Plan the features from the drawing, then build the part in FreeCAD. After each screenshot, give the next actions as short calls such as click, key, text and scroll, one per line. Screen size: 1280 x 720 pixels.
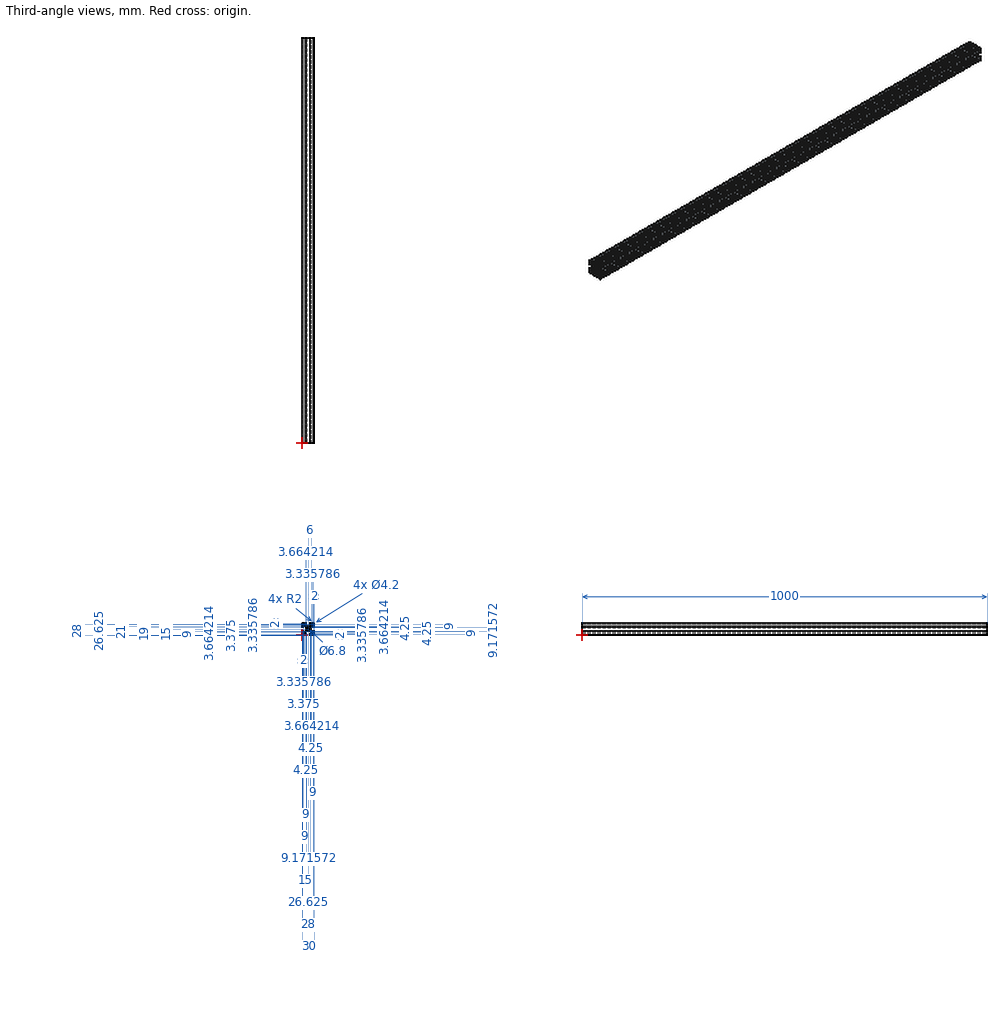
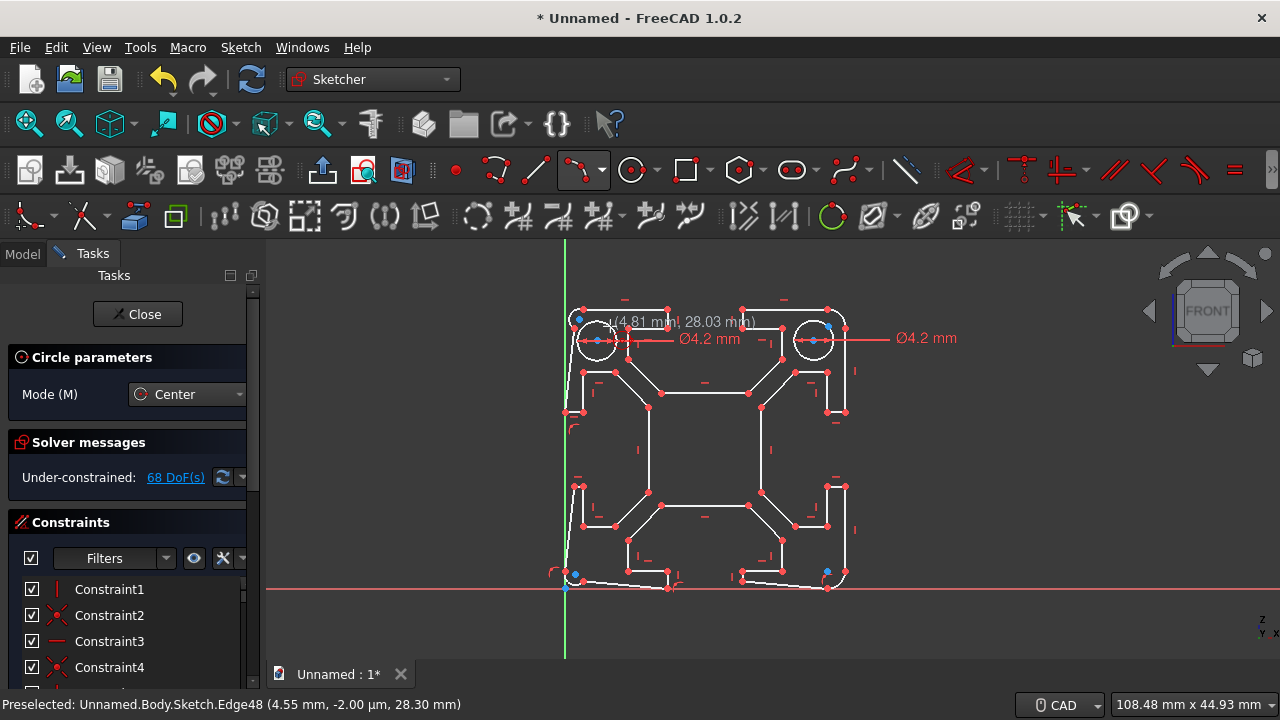
click(814, 557)
move(828, 544)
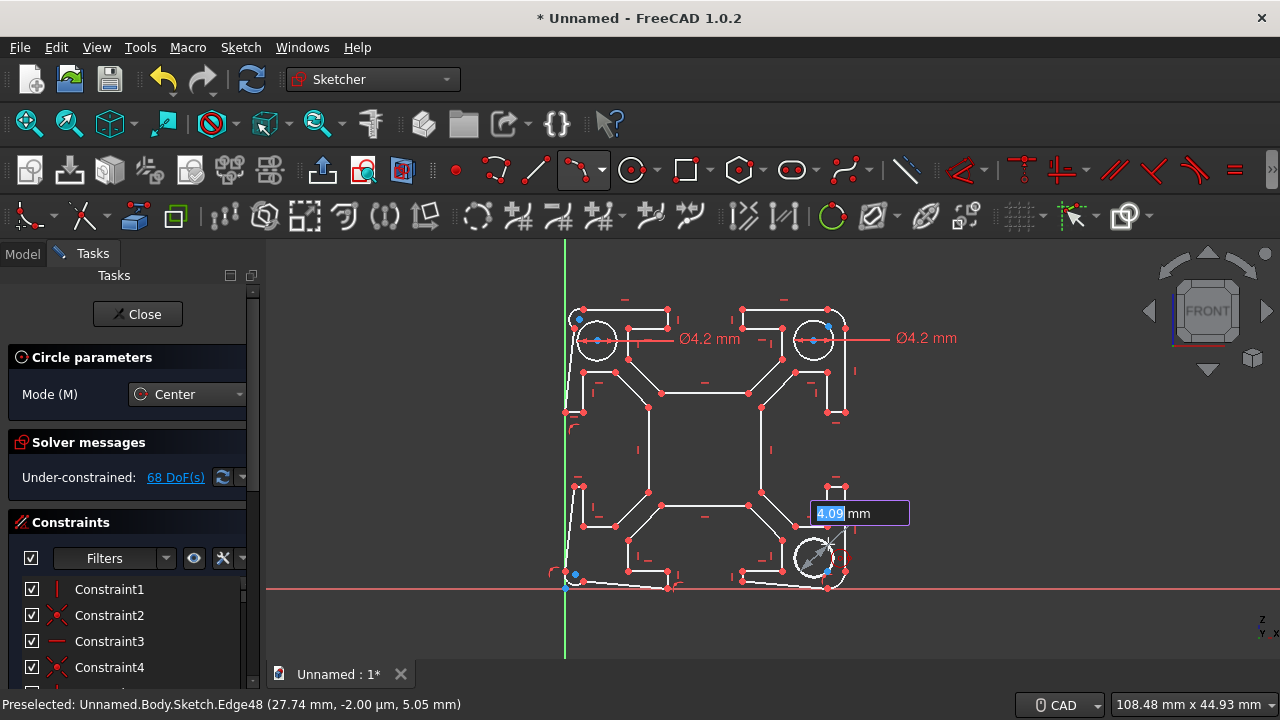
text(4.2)
key(Return)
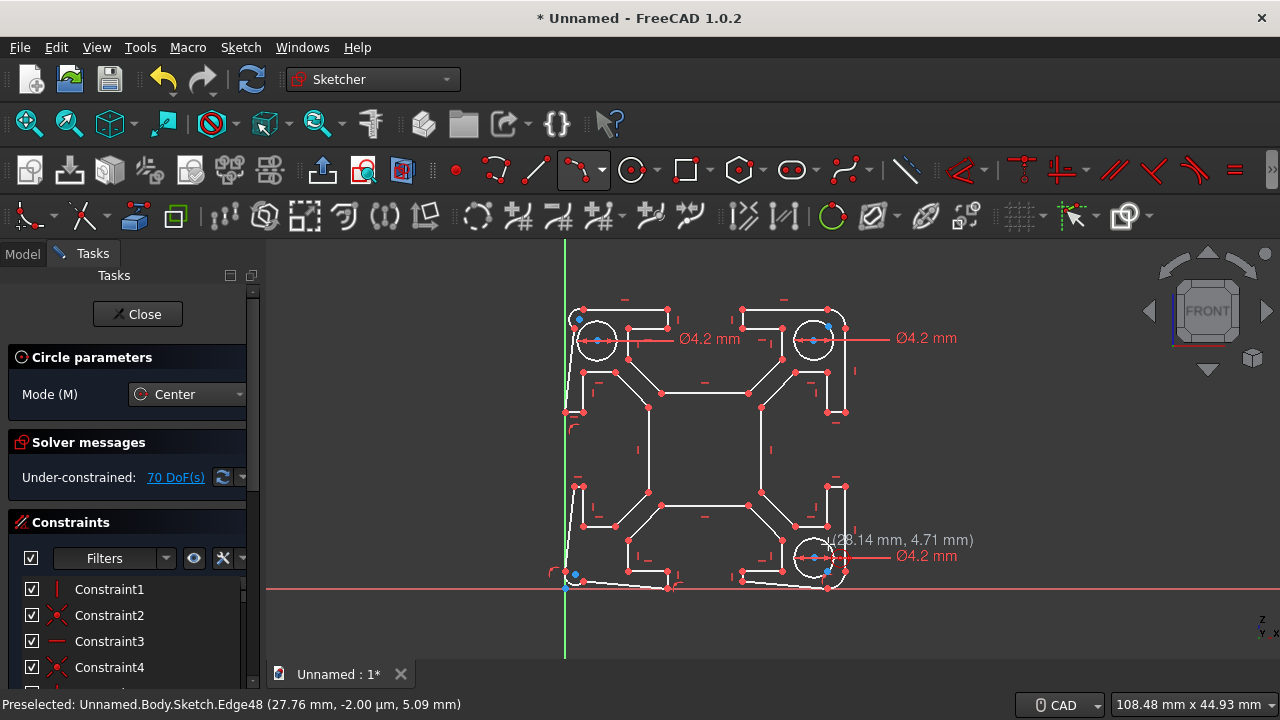
click(705, 449)
move(728, 426)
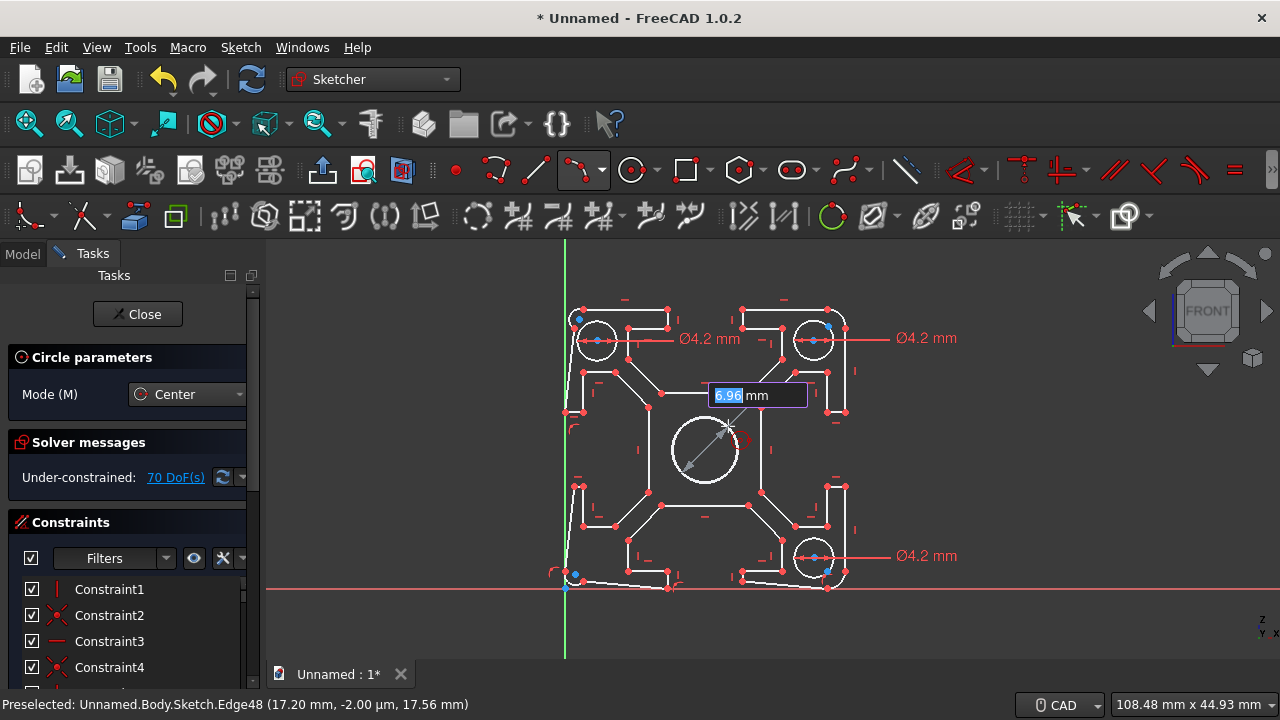
text(6.8)
key(Return)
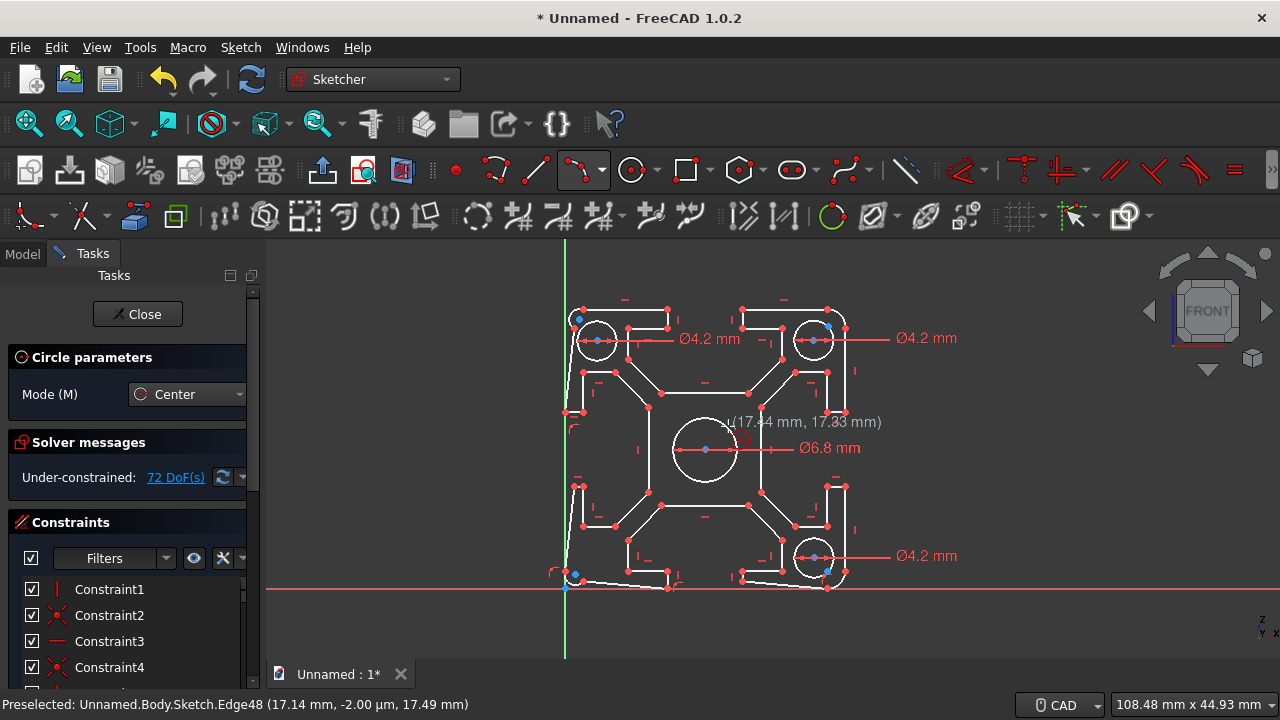
click(597, 557)
move(610, 544)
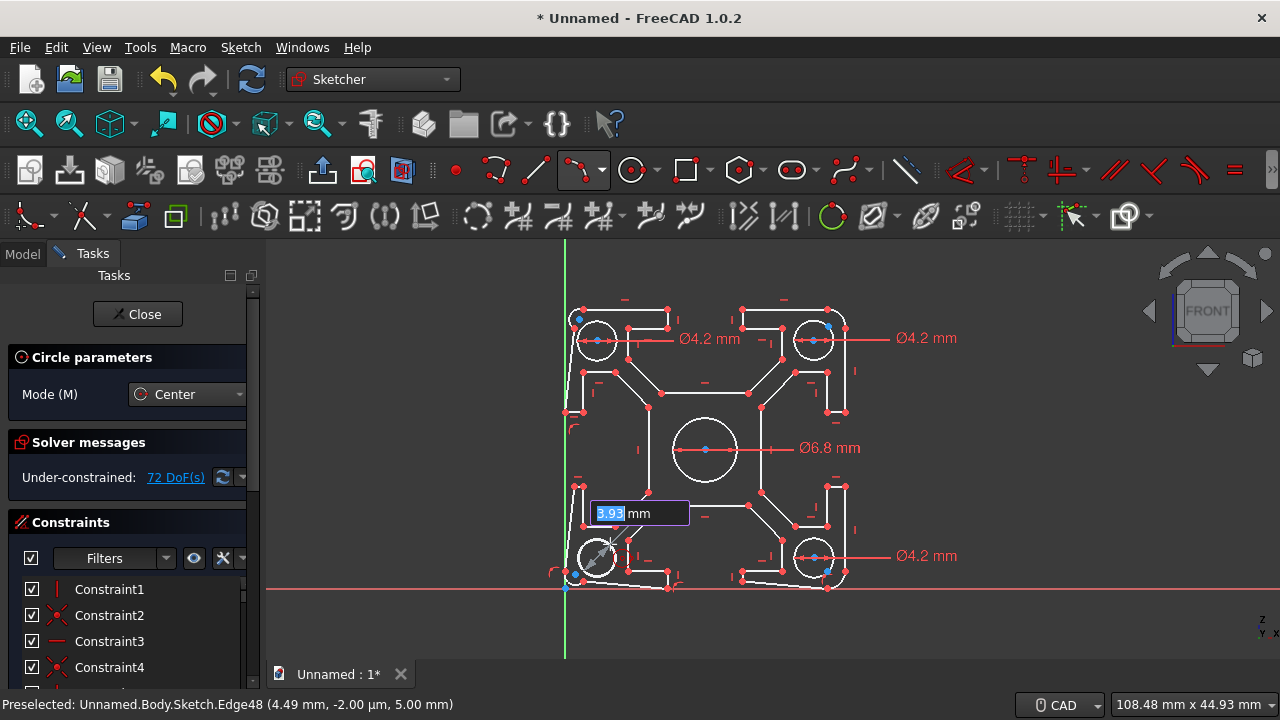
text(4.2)
key(Return)
key(Escape)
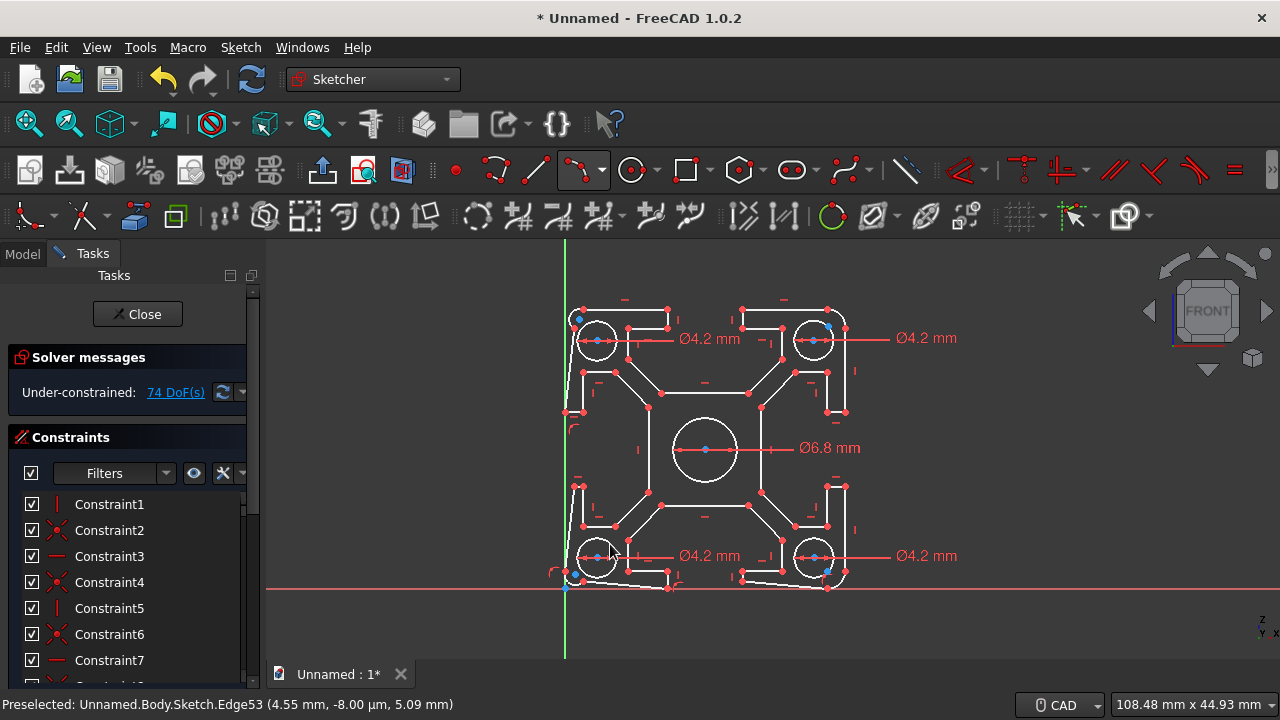
click(845, 354)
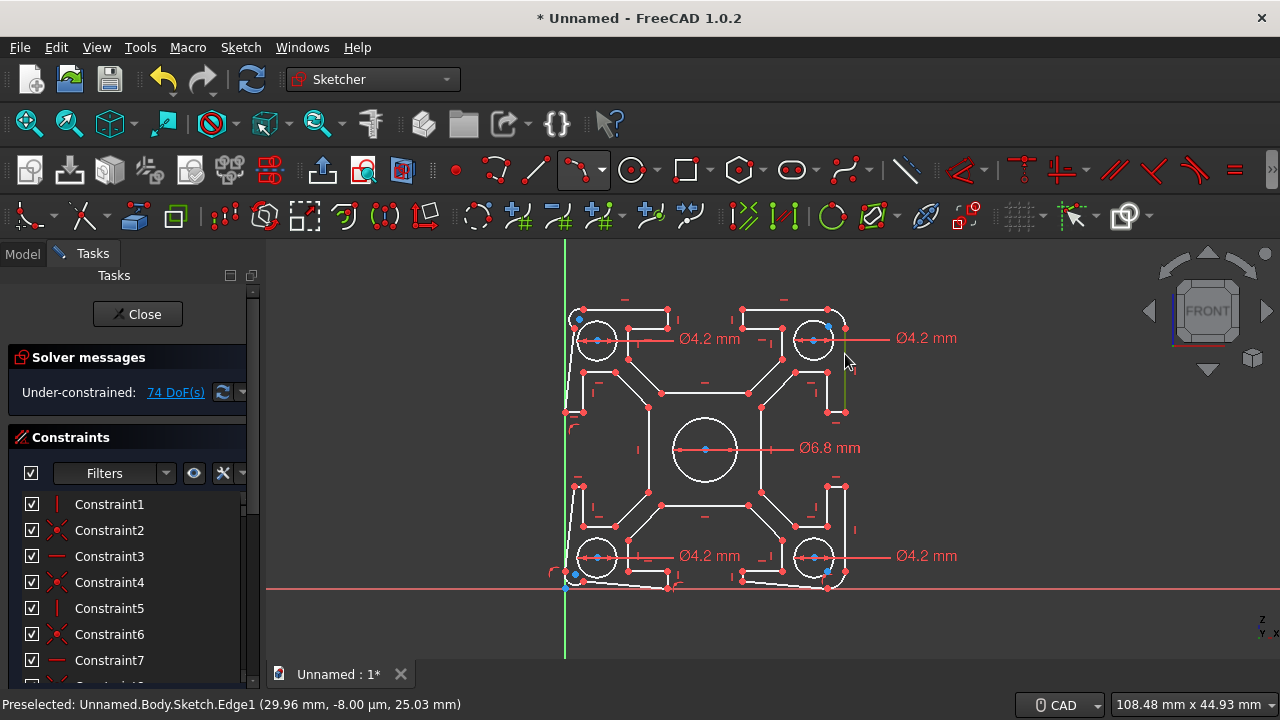
click(841, 315)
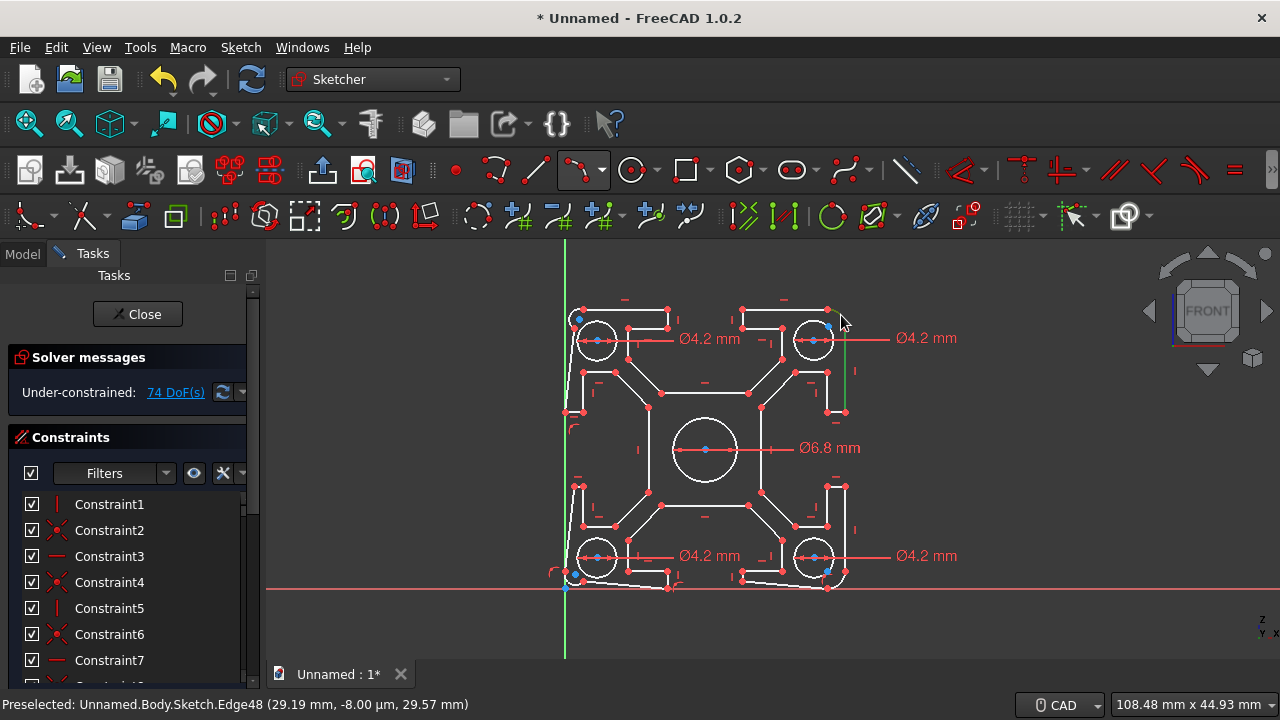
click(1196, 170)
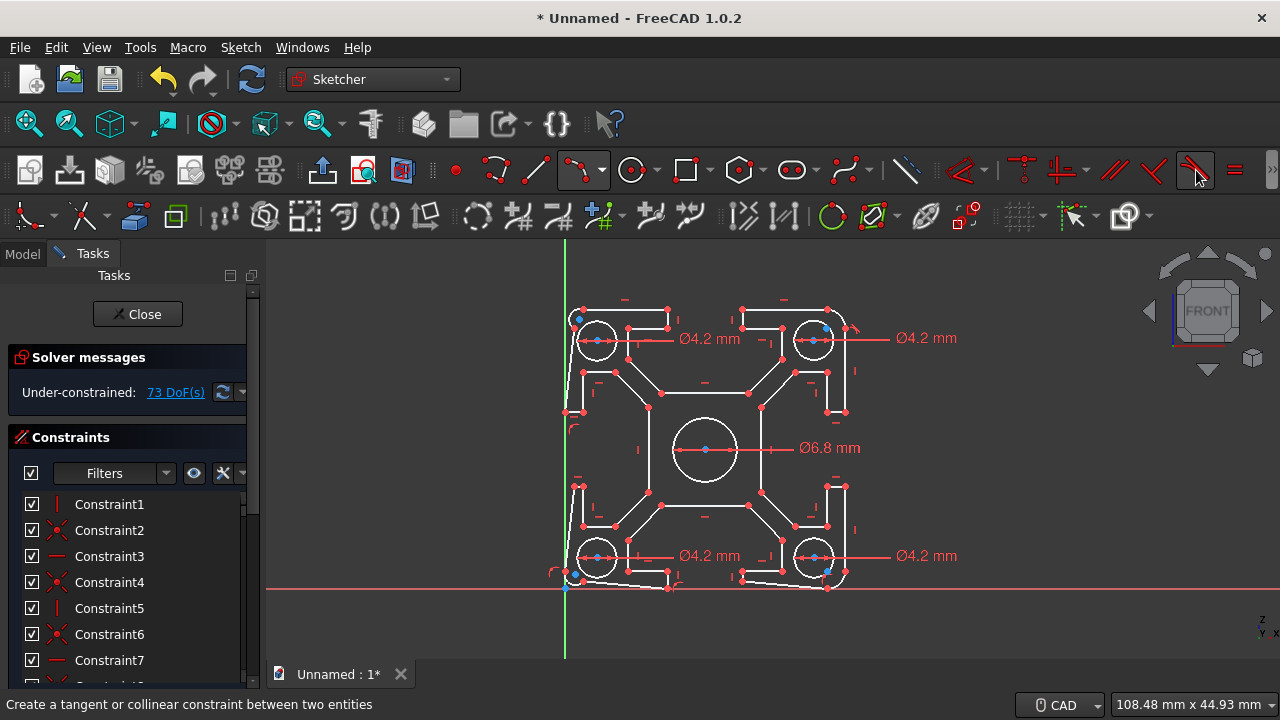
click(845, 512)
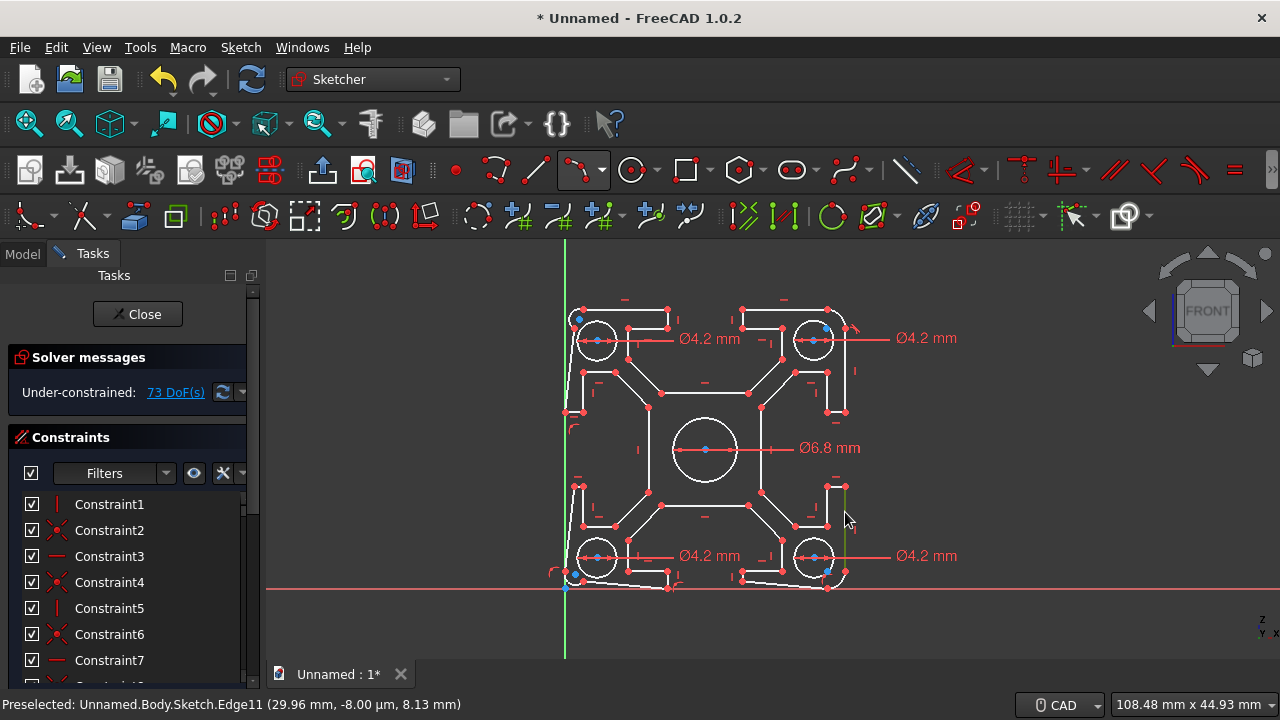
scroll(835, 587, up, 3)